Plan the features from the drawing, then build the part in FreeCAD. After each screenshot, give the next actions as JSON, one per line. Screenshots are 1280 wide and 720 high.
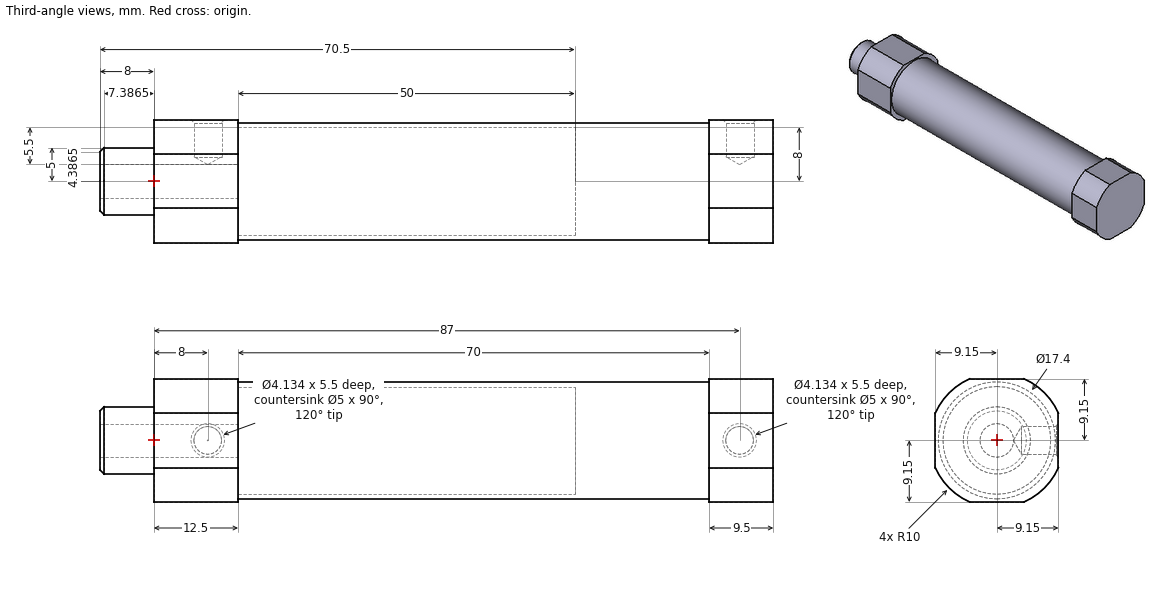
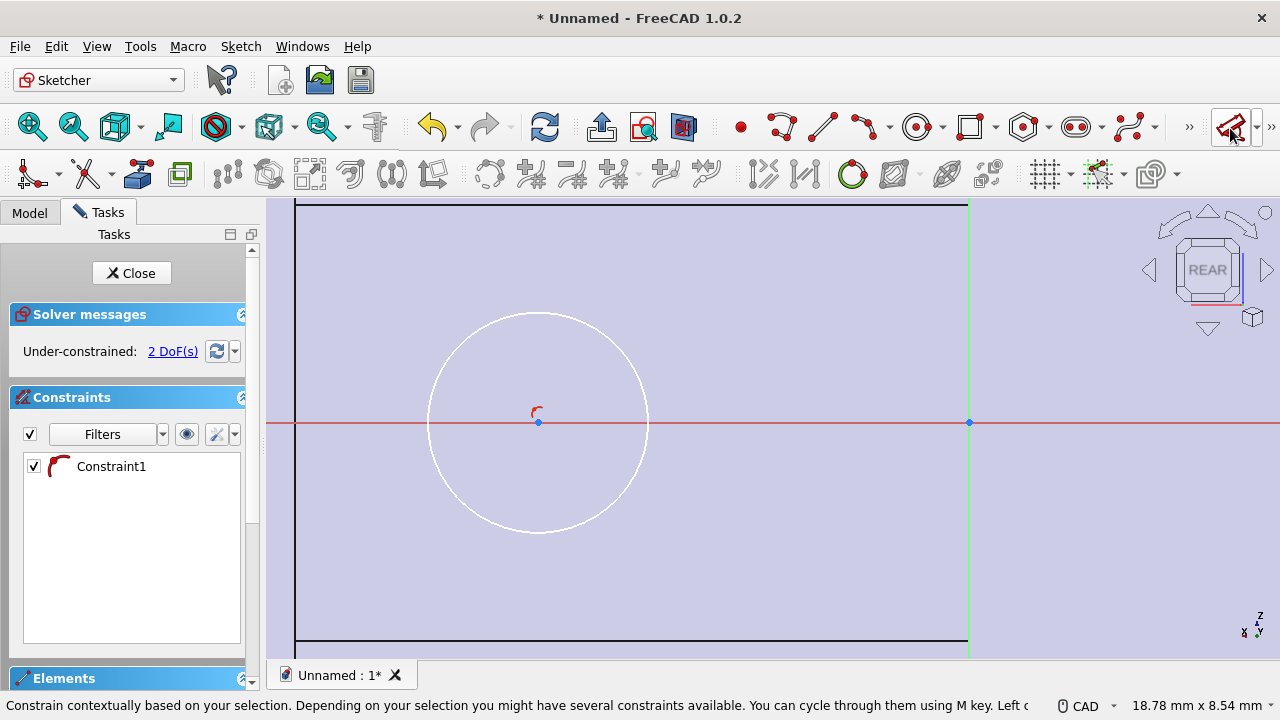
{"action": "left_click", "coordinate": [616, 345]}
{"action": "left_click", "coordinate": [639, 322]}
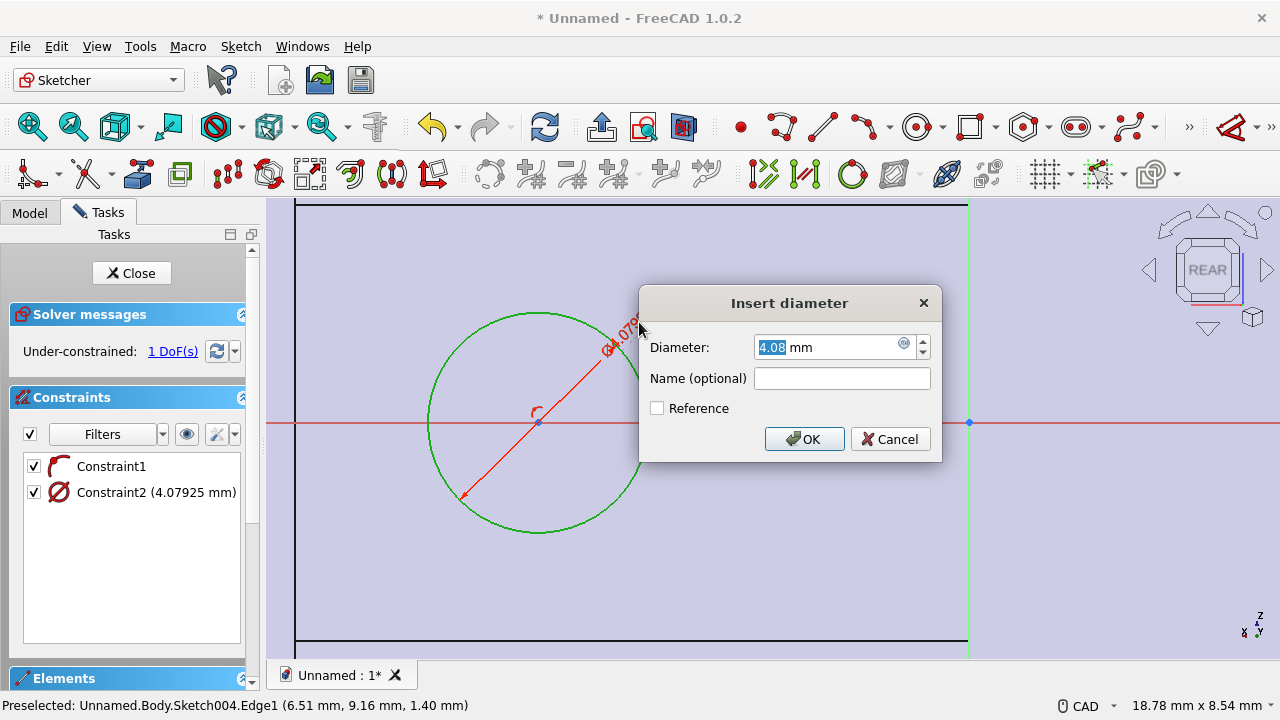
{"action": "type", "text": "4.134"}
{"action": "key", "text": "Return"}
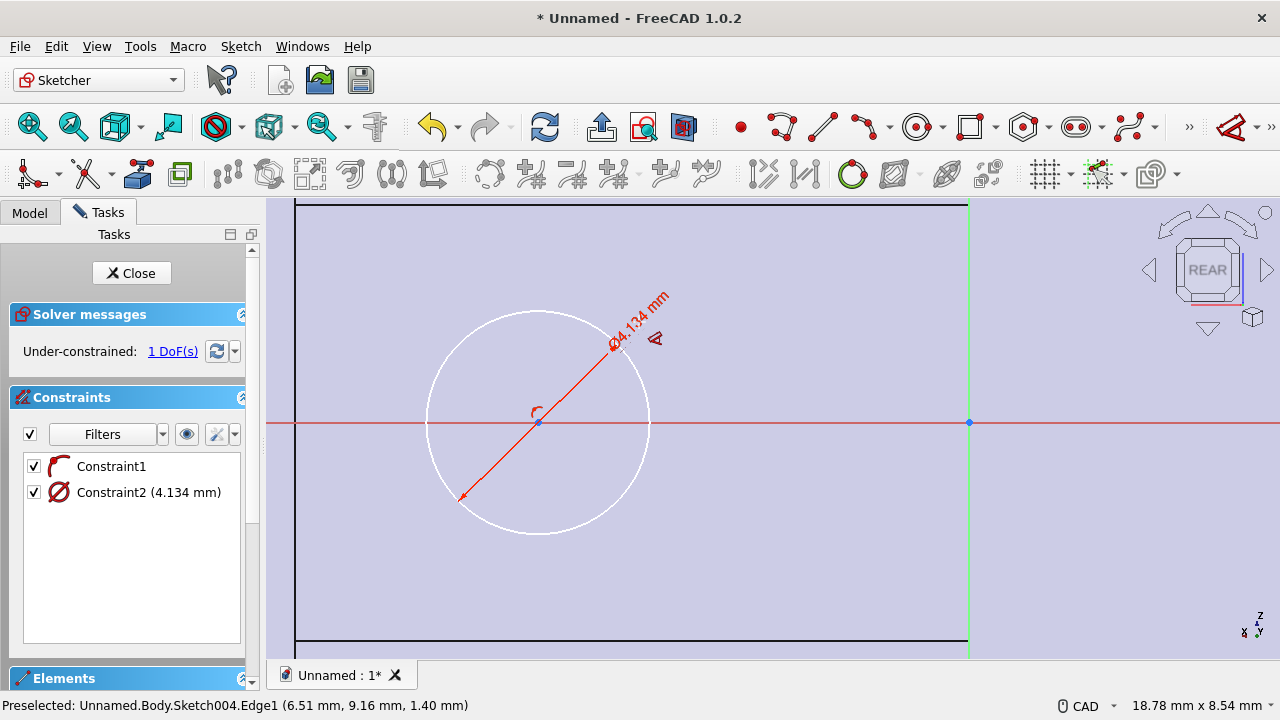
{"action": "left_click", "coordinate": [538, 423]}
{"action": "left_click", "coordinate": [754, 457]}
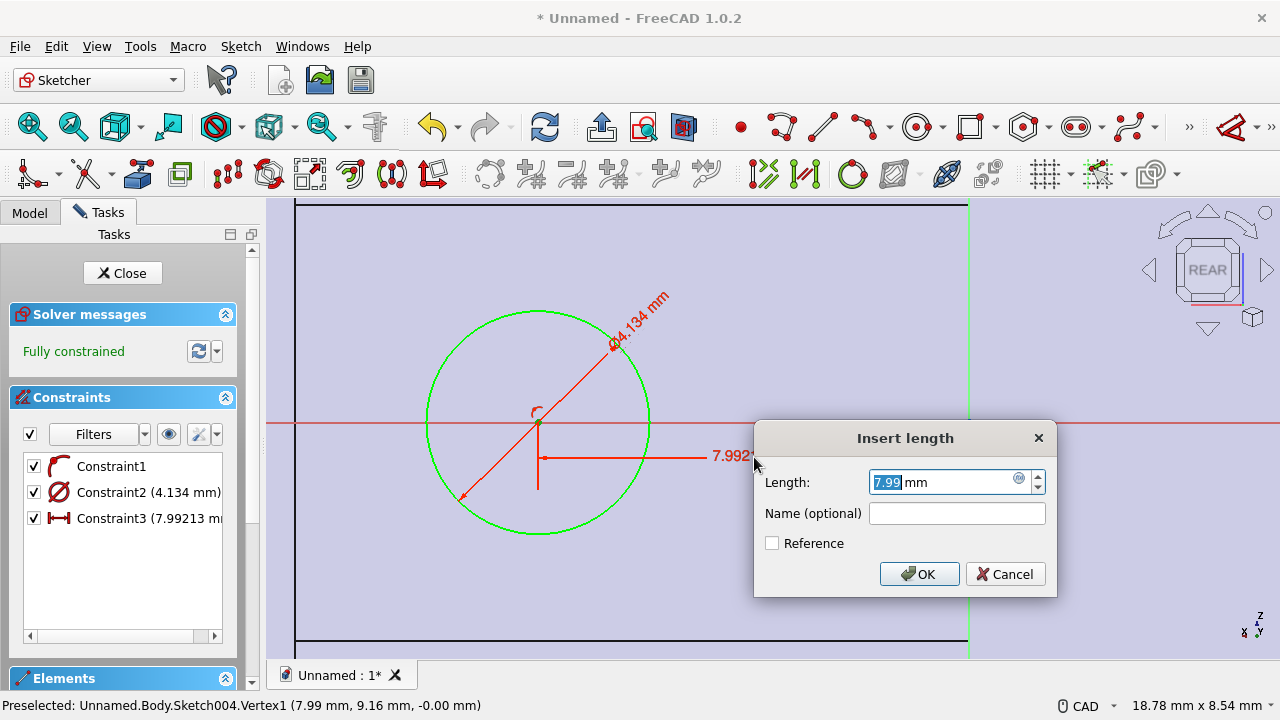
{"action": "type", "text": "8"}
{"action": "key", "text": "Return"}
{"action": "key", "text": "Escape"}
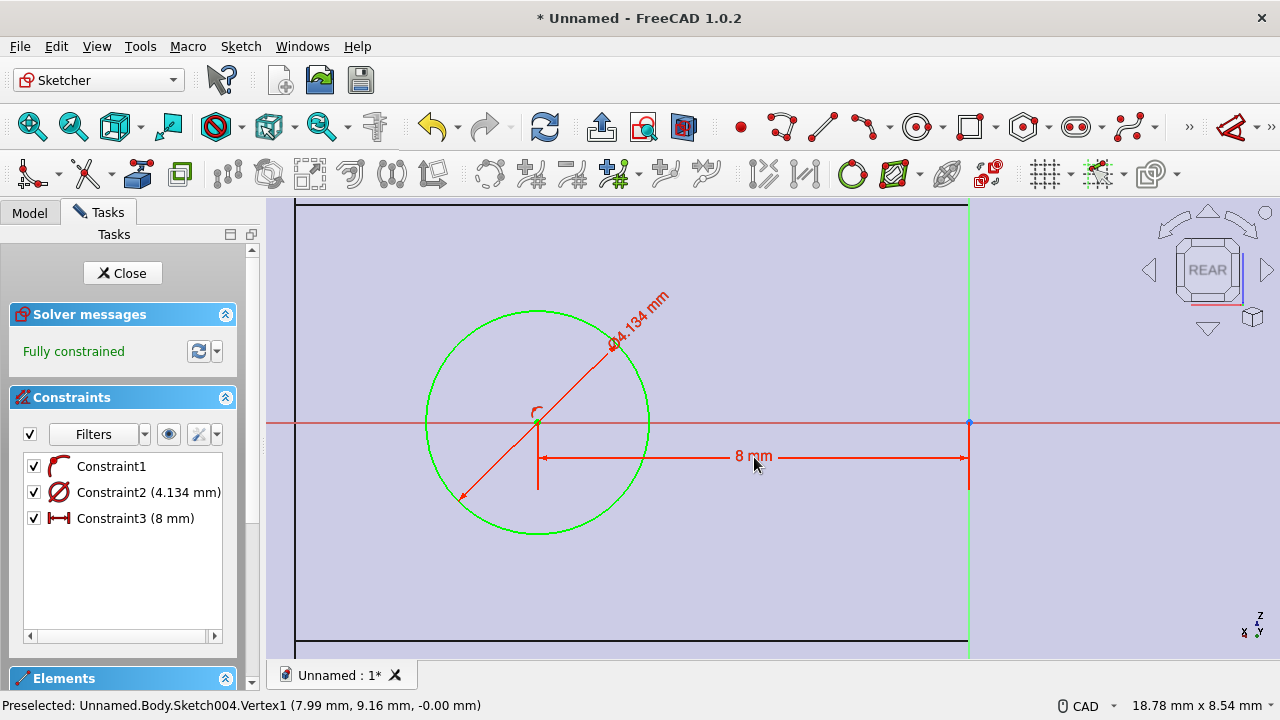
{"action": "left_click", "coordinate": [123, 273]}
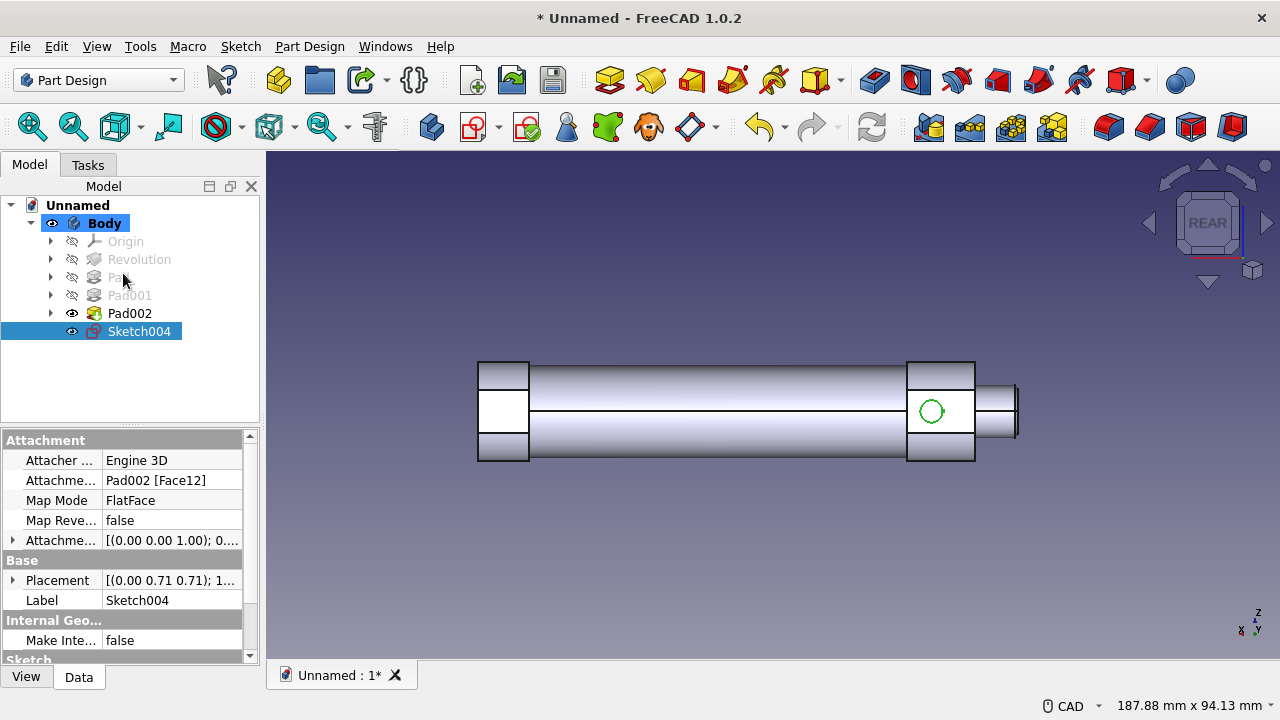
{"action": "left_click", "coordinate": [916, 80]}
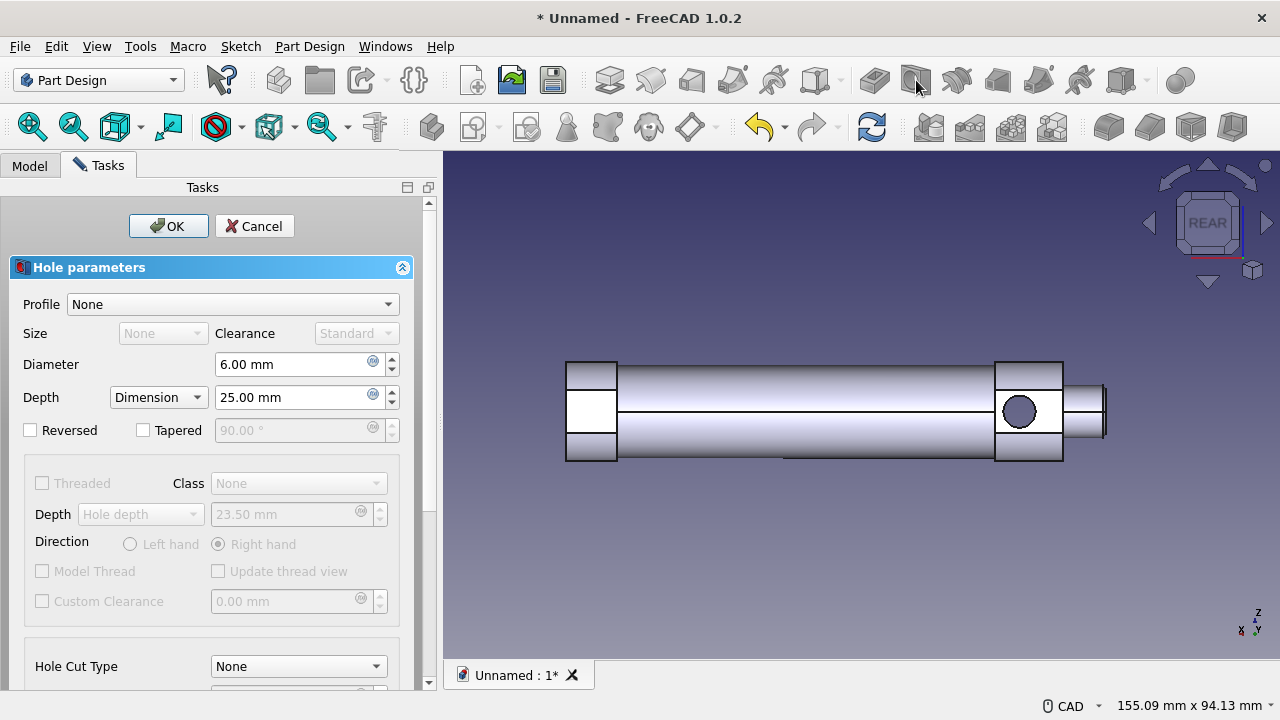
{"action": "triple_click", "coordinate": [300, 364]}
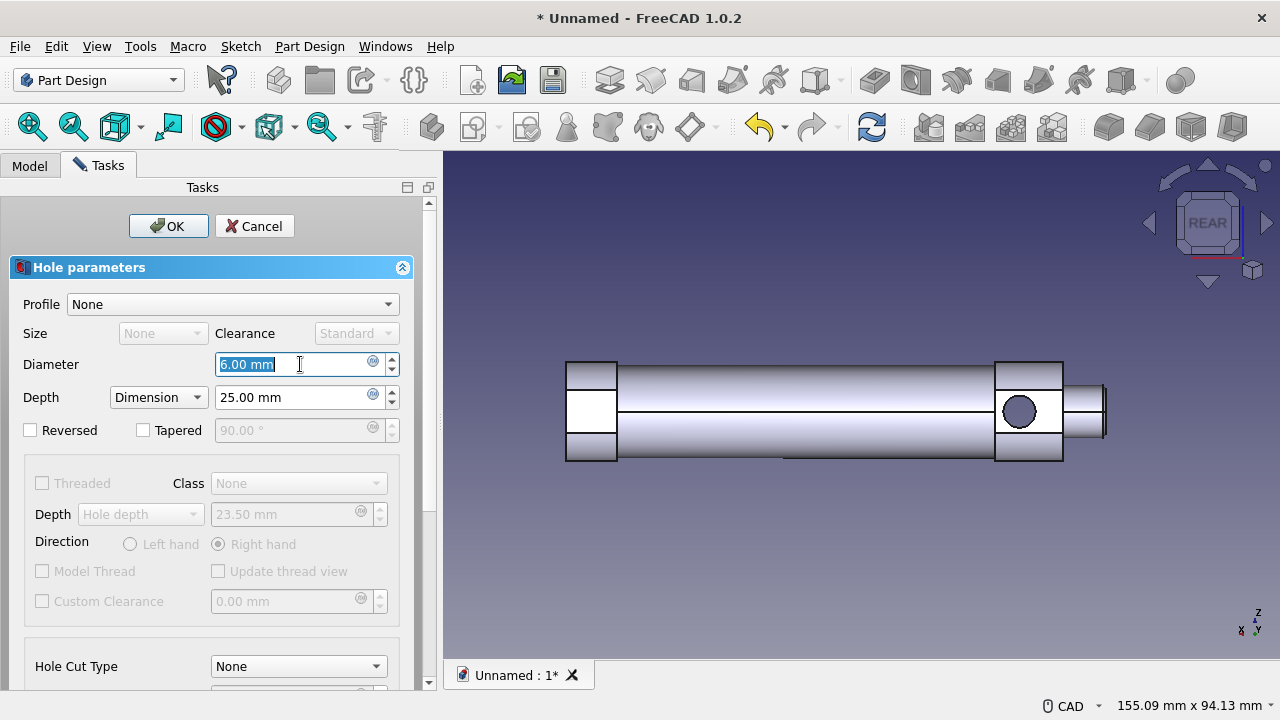
{"action": "type", "text": "4.134"}
{"action": "key", "text": "Tab"}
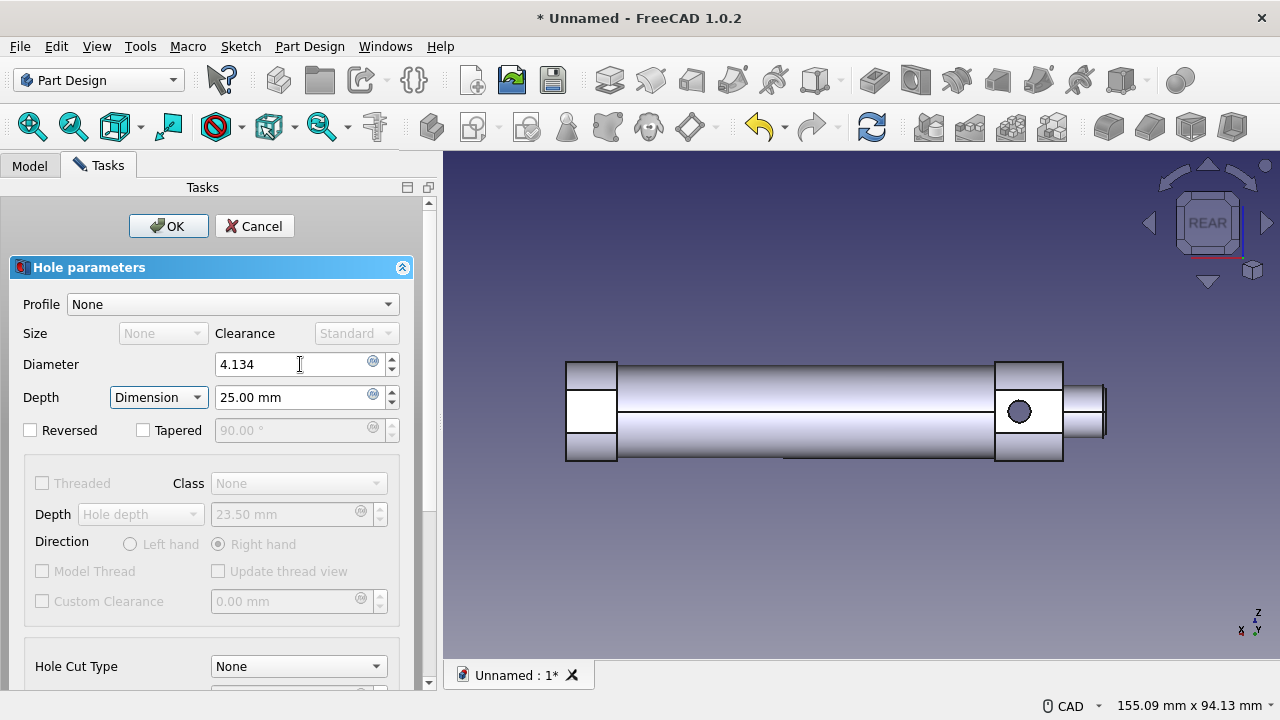
{"action": "triple_click", "coordinate": [300, 398]}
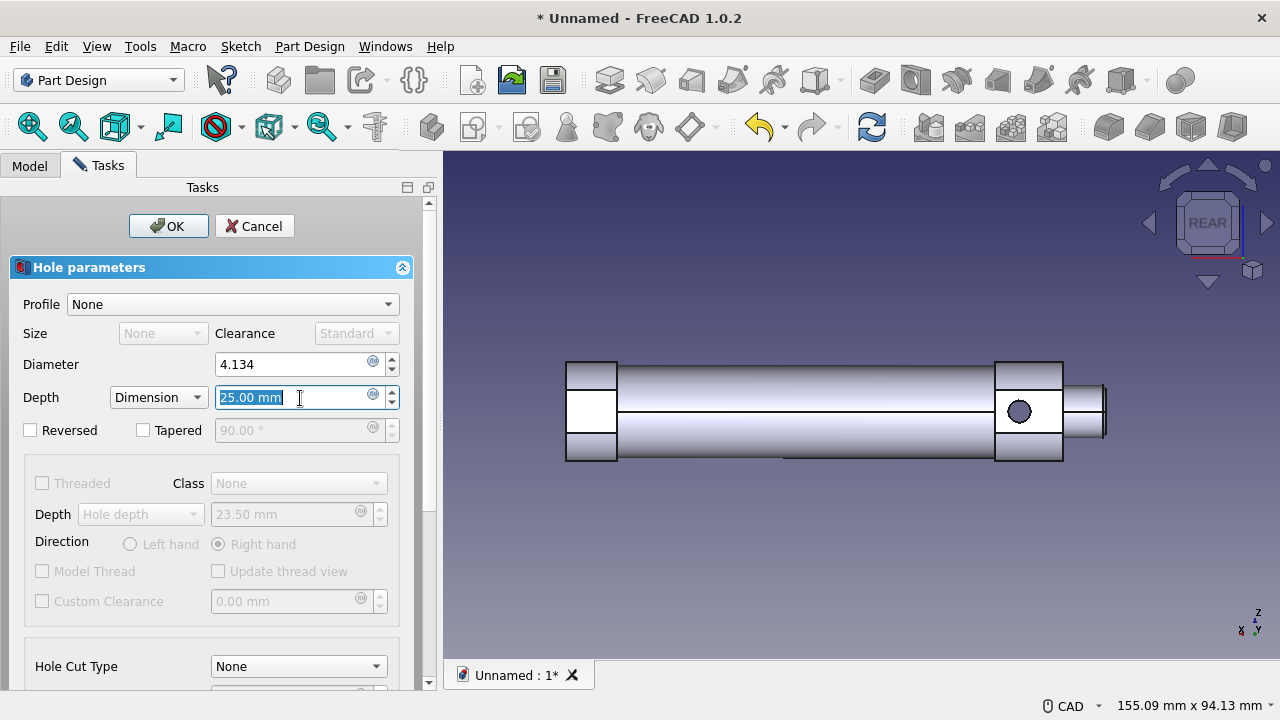
{"action": "type", "text": "5.5"}
{"action": "key", "text": "Tab"}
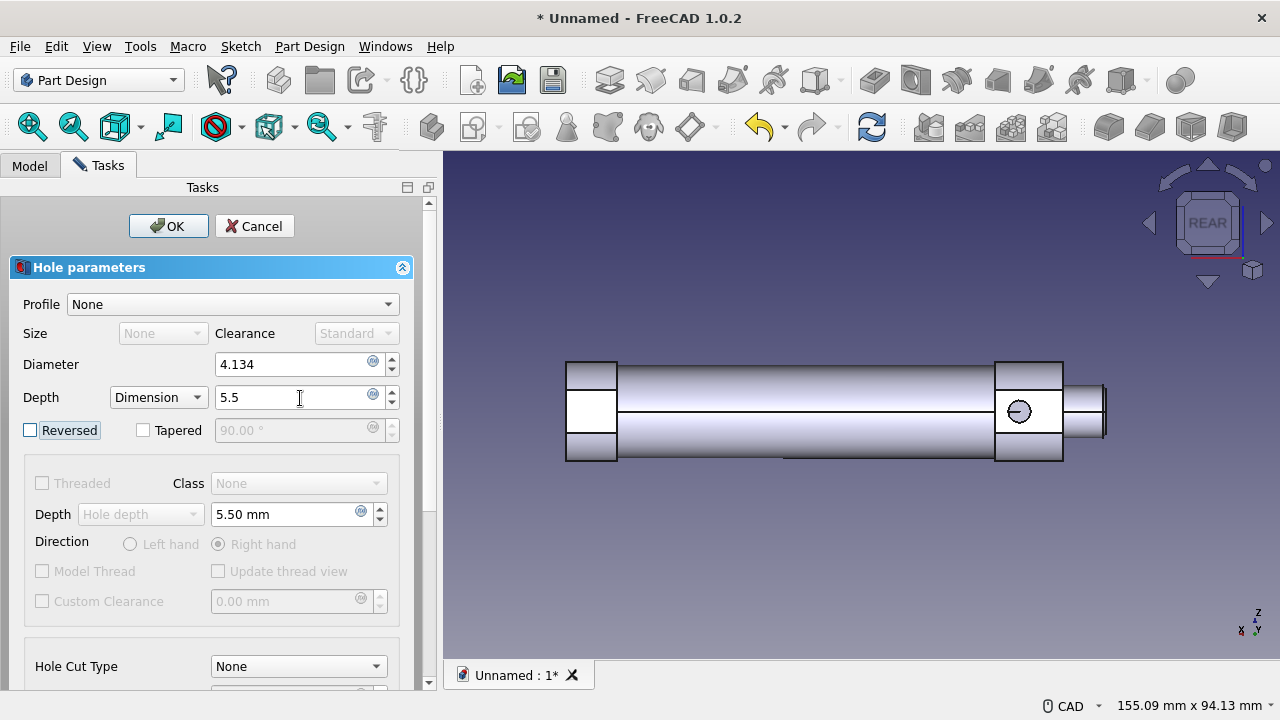
{"action": "left_click", "coordinate": [300, 666]}